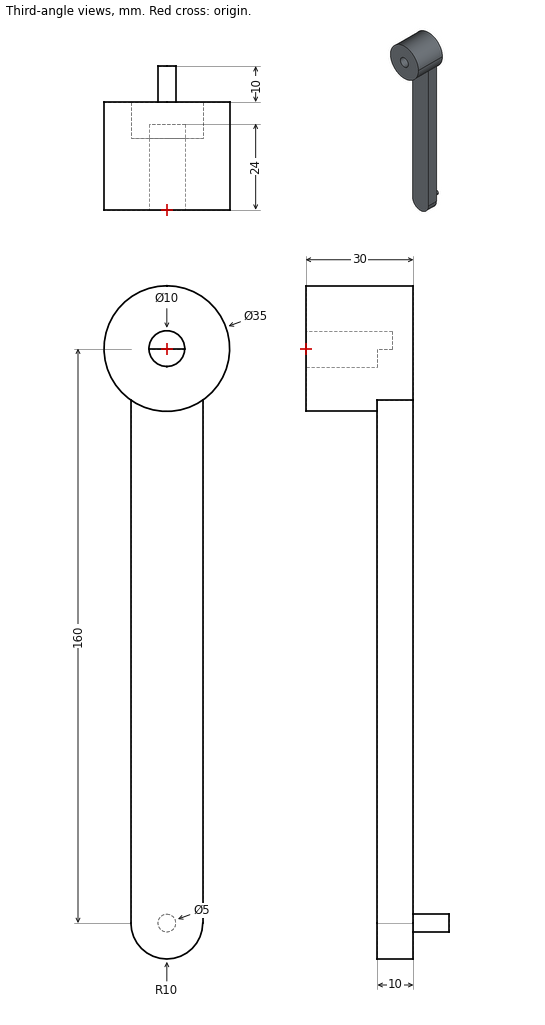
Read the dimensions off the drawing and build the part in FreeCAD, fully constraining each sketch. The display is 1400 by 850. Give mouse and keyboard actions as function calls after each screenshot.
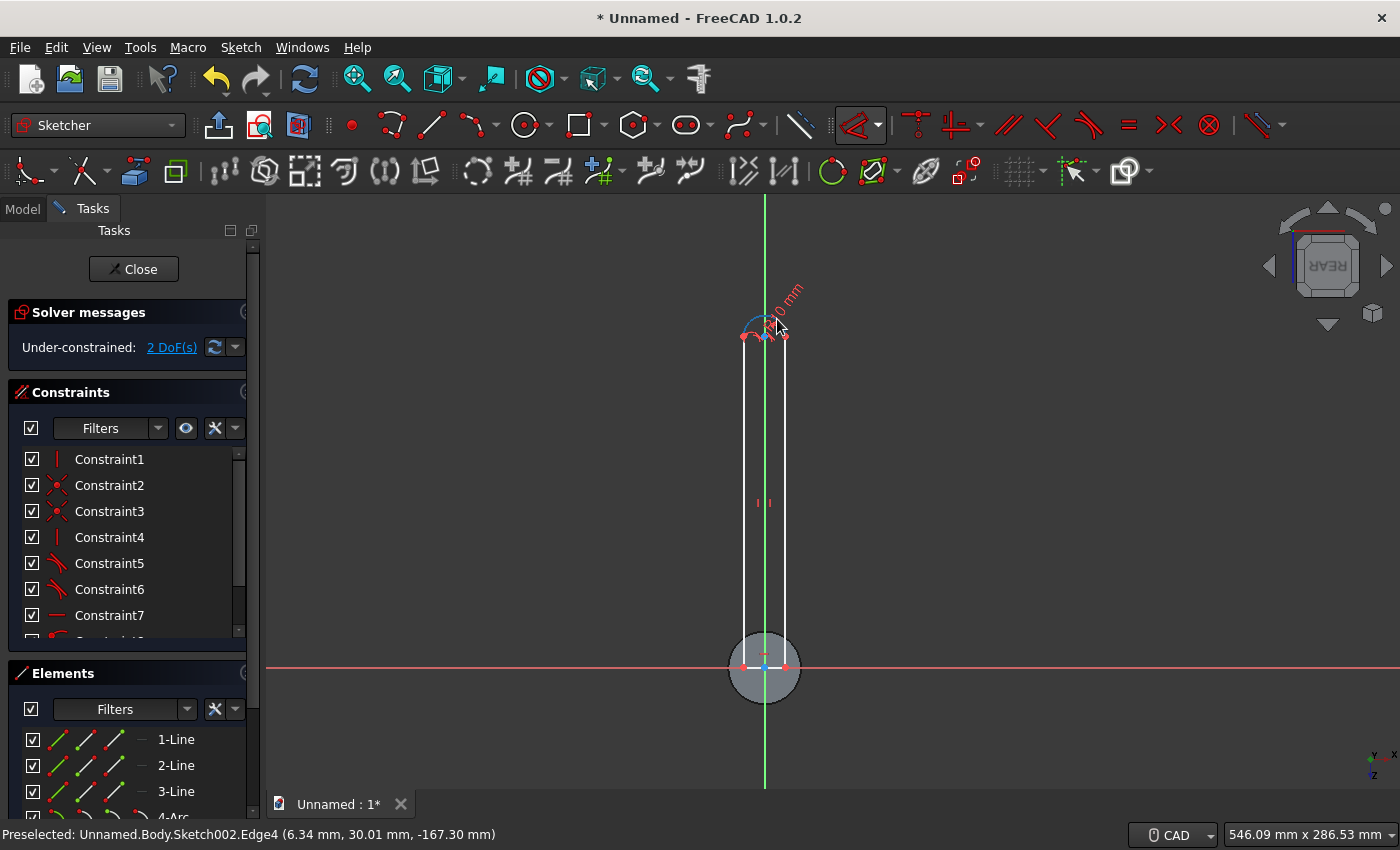
click(744, 668)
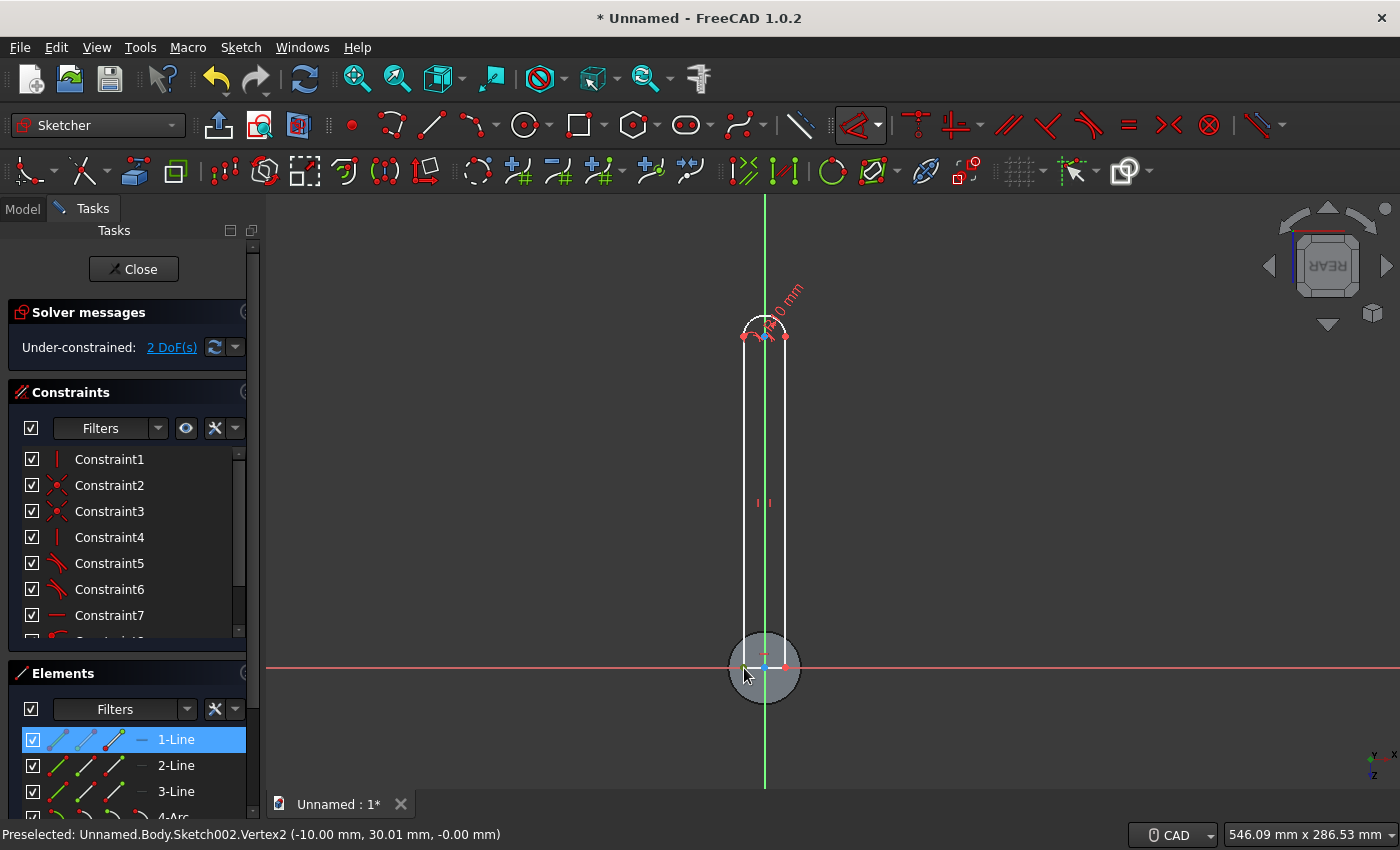
click(361, 668)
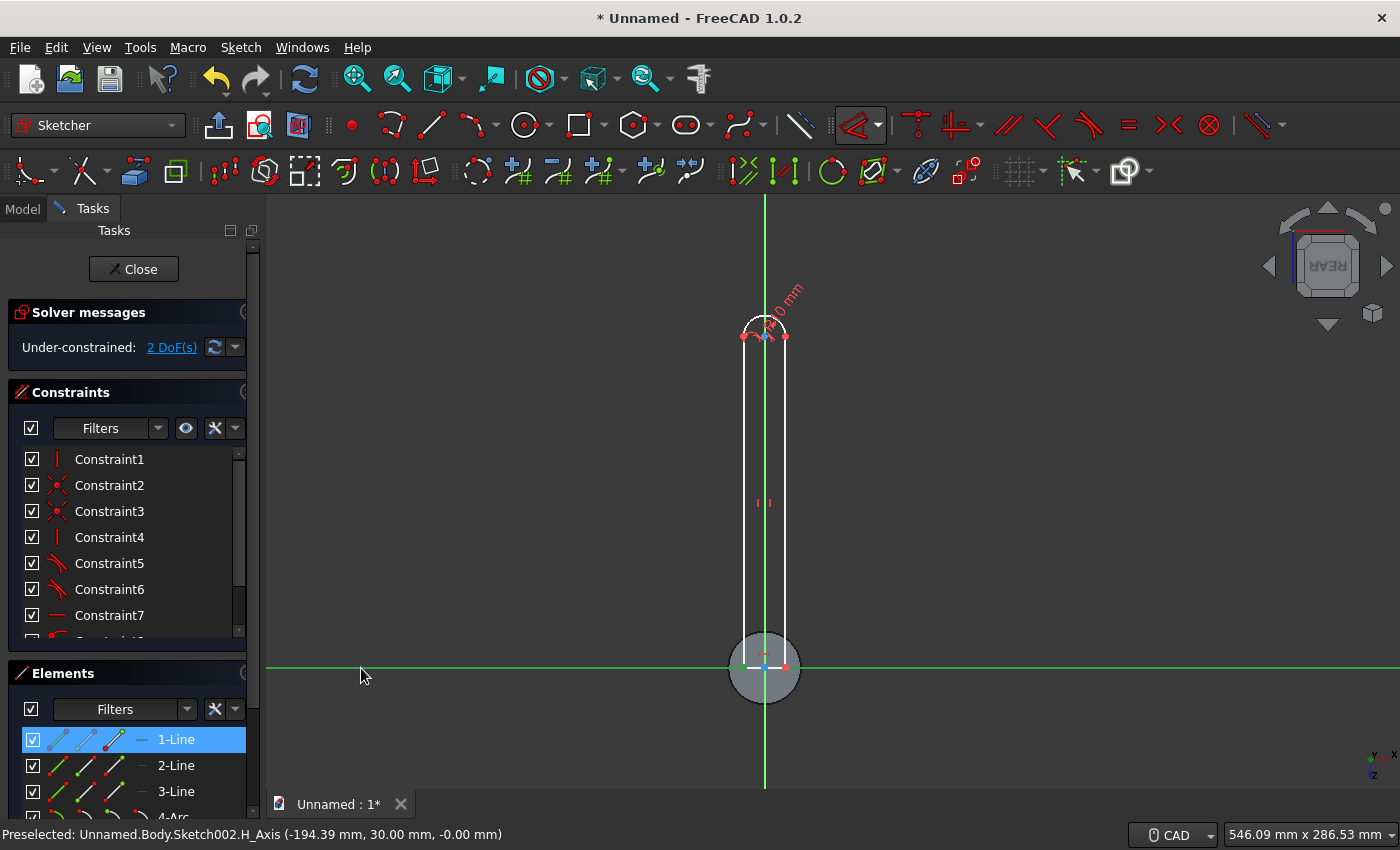
key(c)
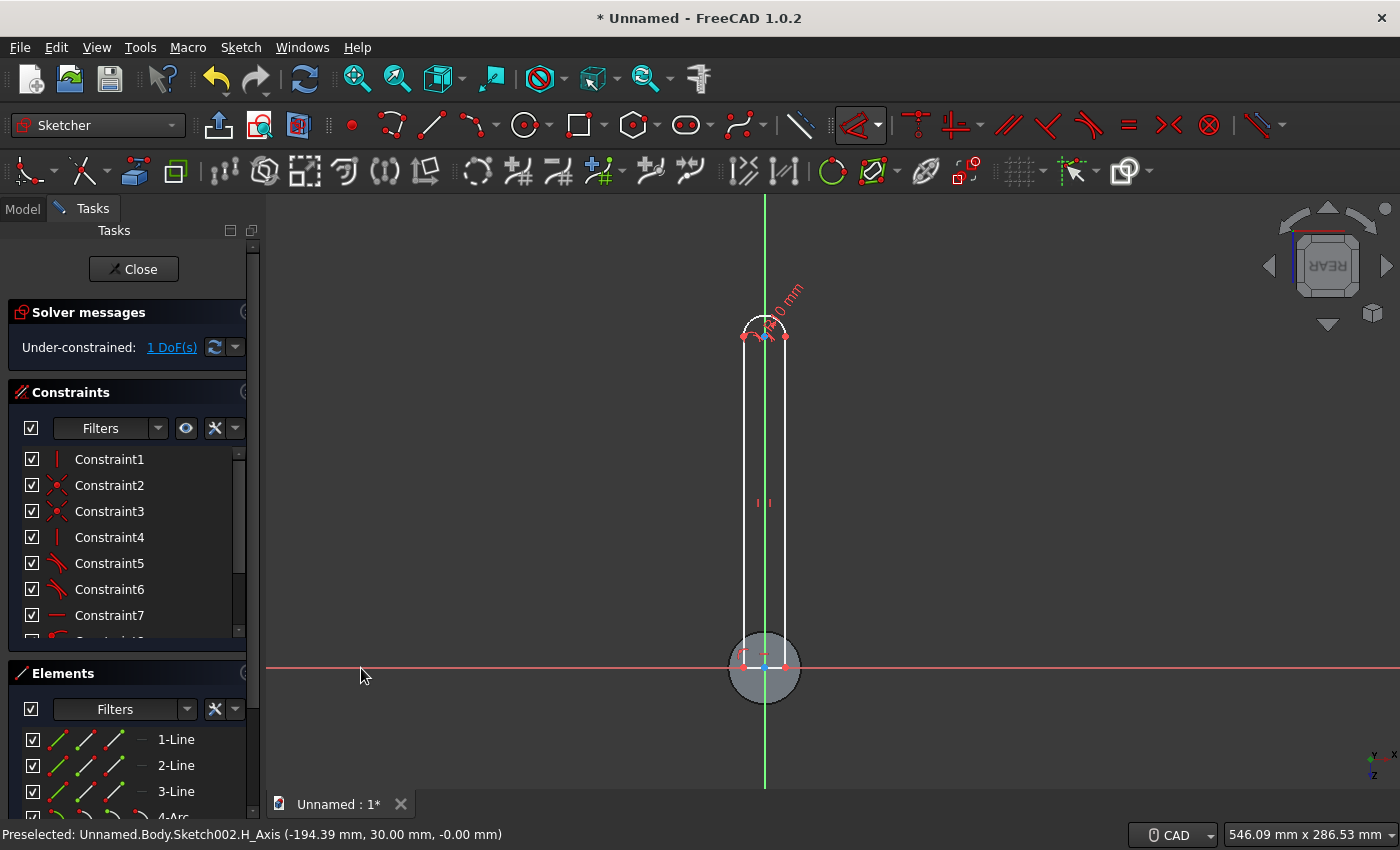
key(d)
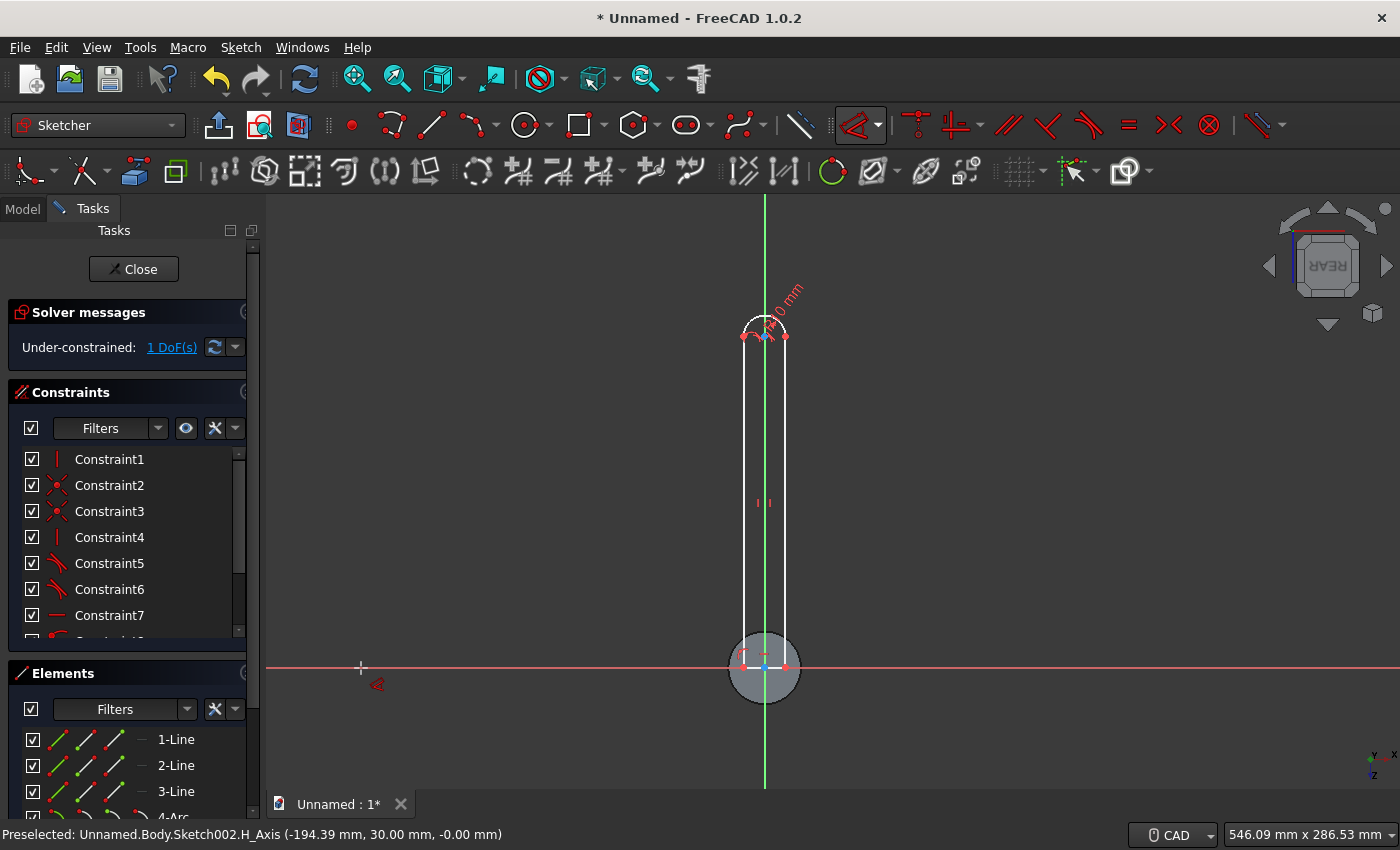
click(744, 436)
click(710, 502)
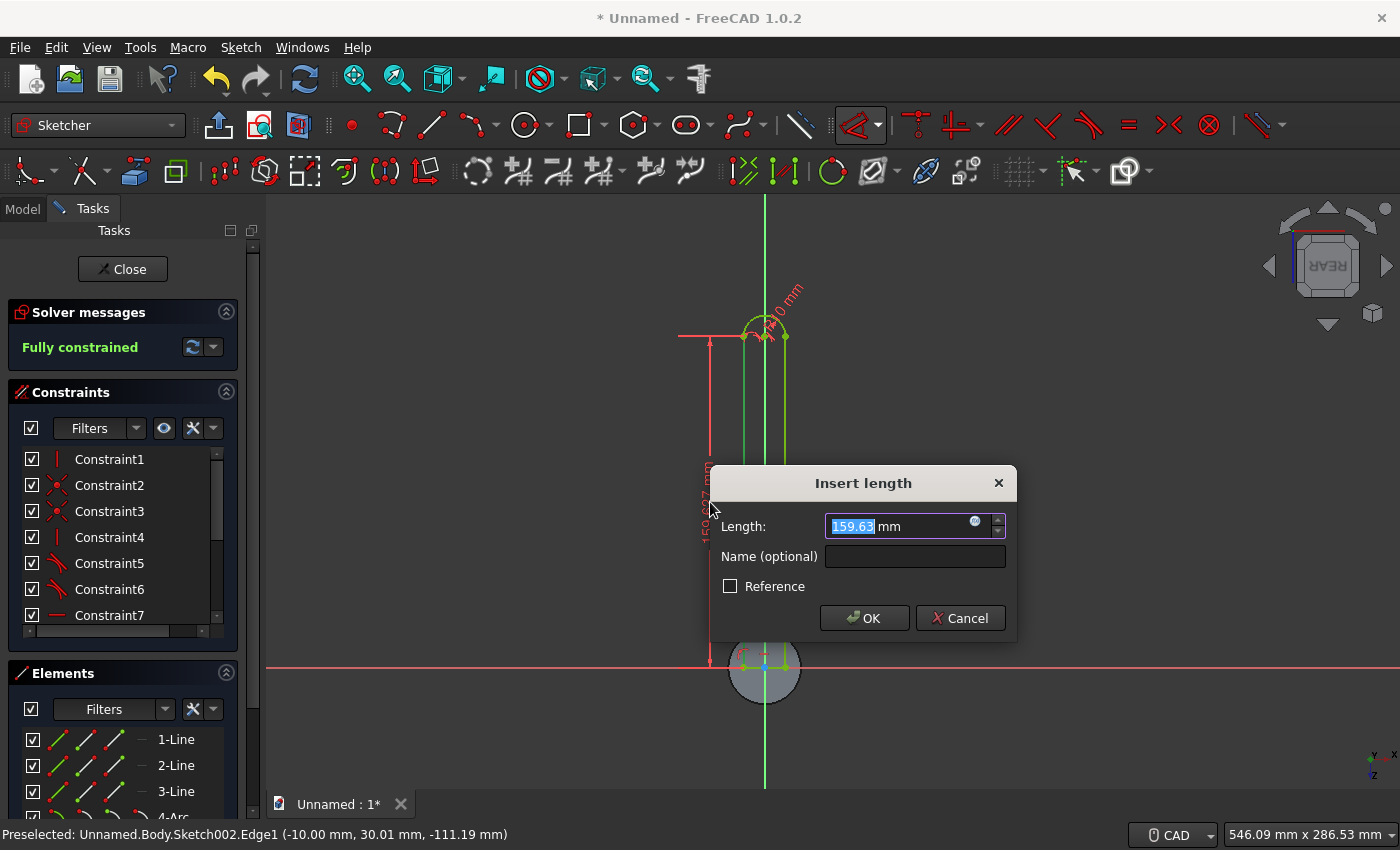
text(160)
key(Return)
key(Escape)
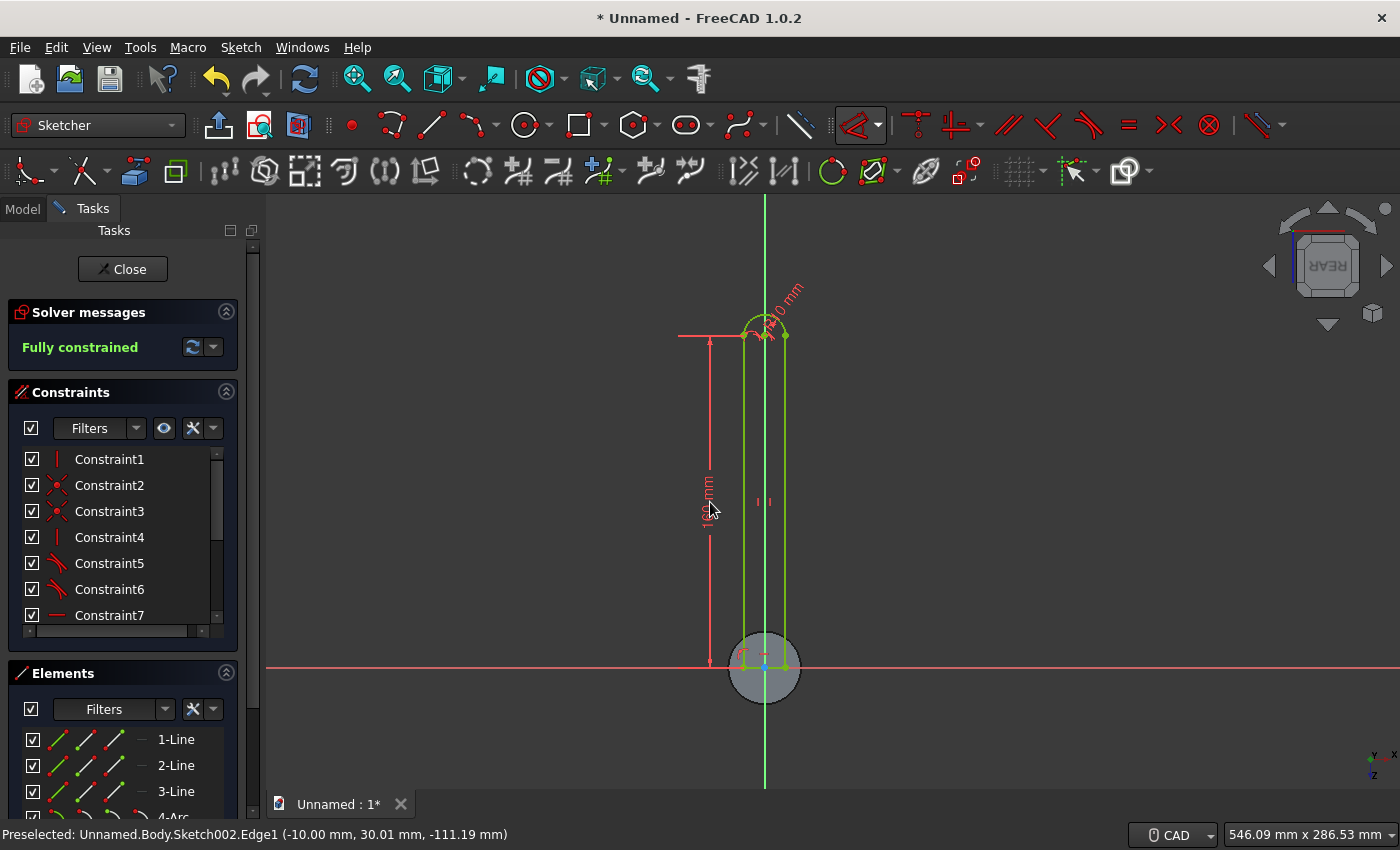
click(123, 269)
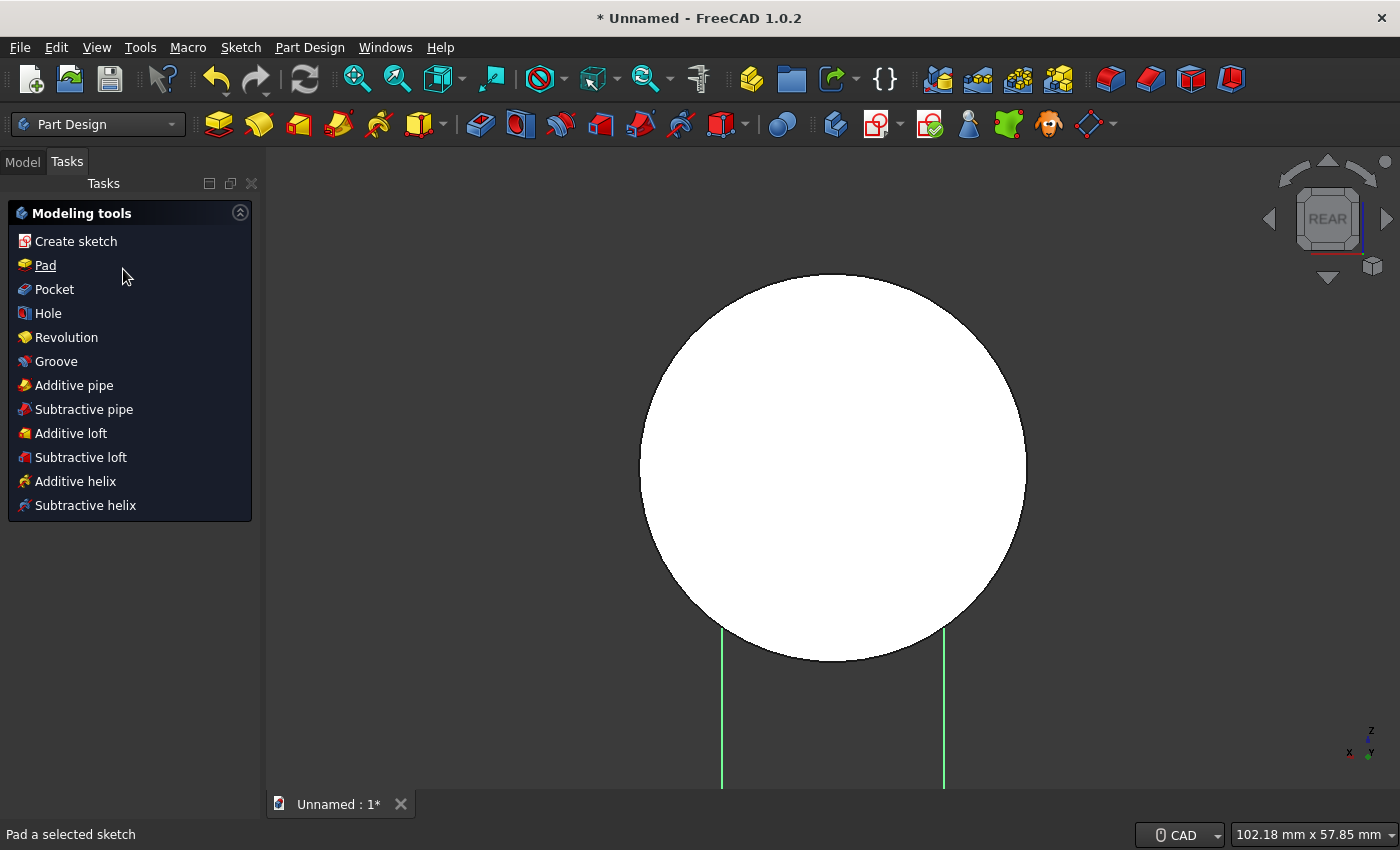
click(220, 124)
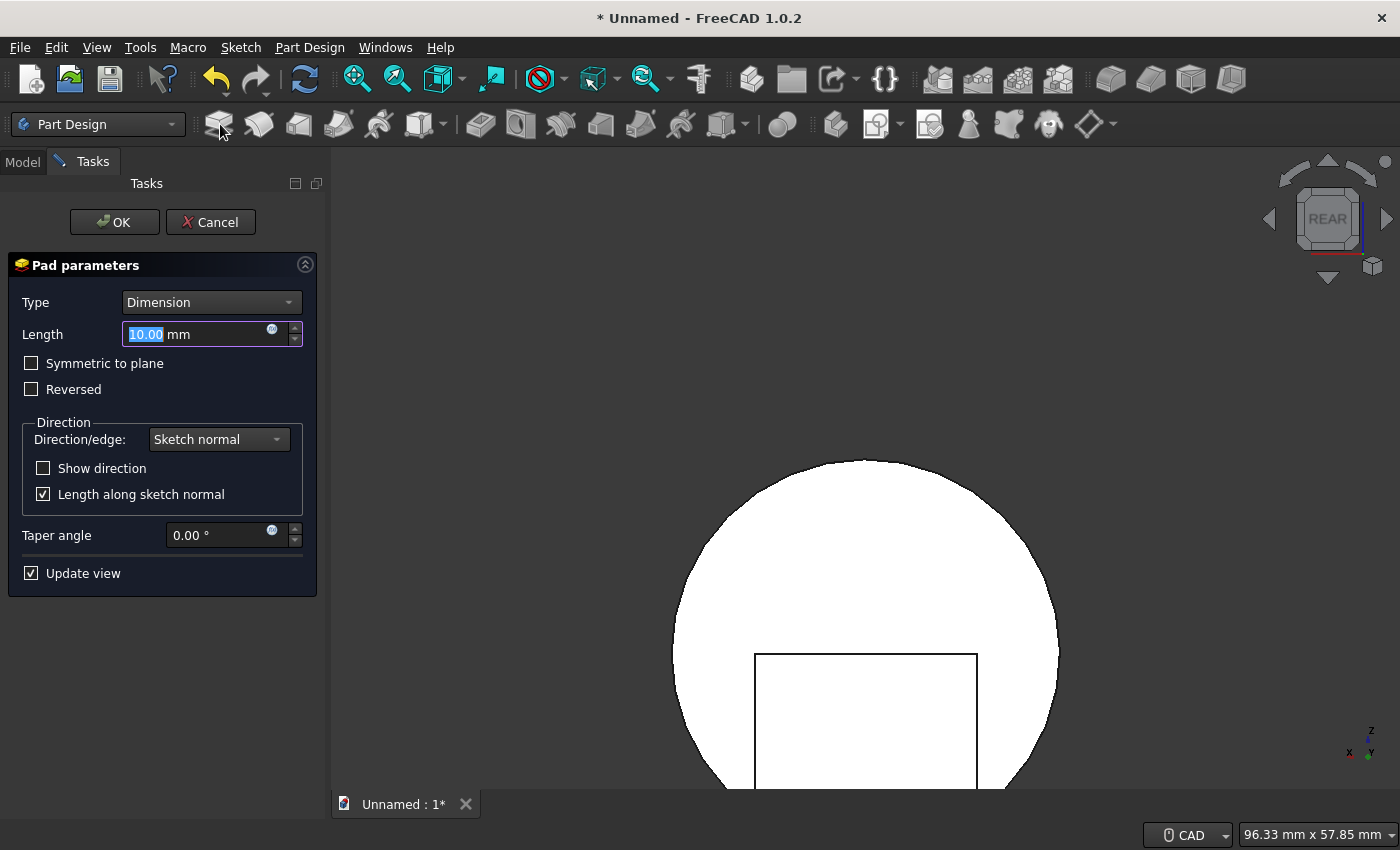
text(10)
key(Tab)